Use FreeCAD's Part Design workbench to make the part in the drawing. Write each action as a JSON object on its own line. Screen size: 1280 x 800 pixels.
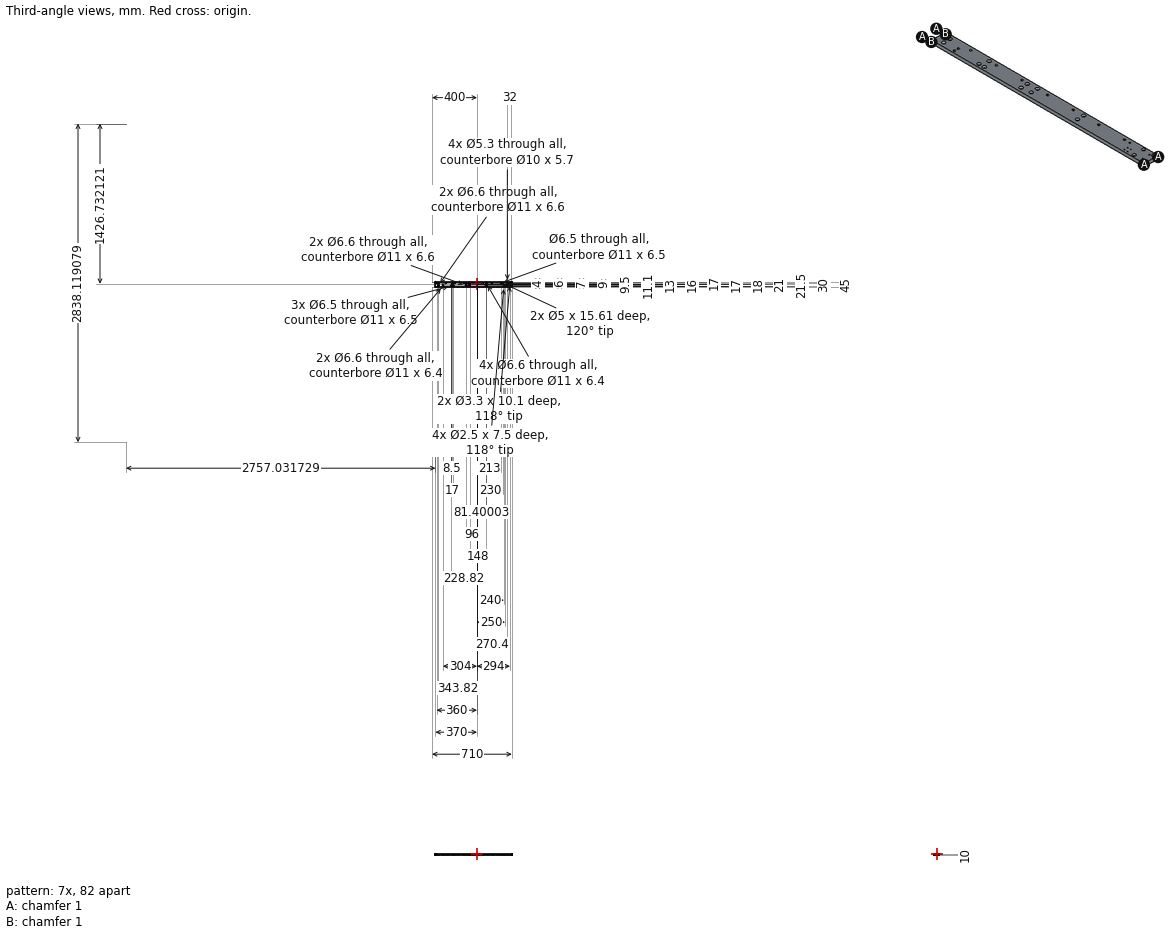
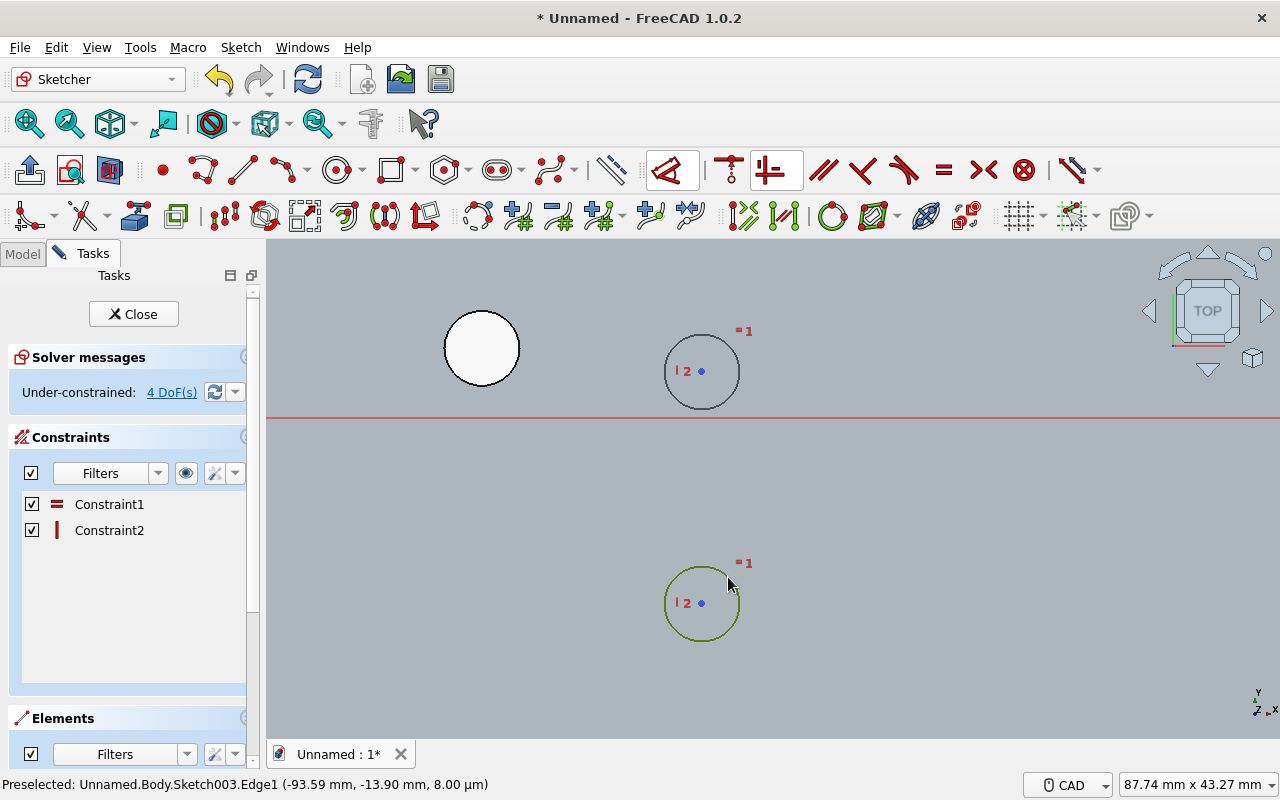
{"action": "key", "text": "k o"}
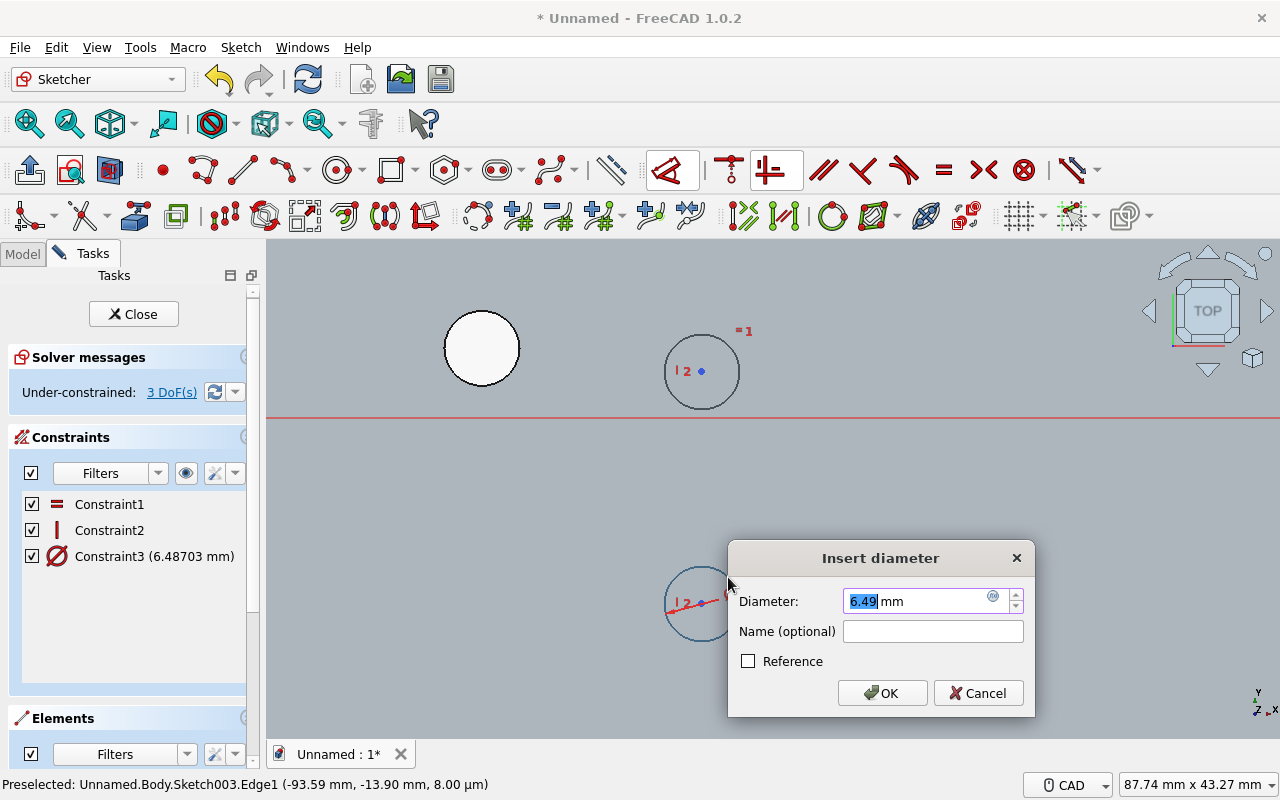
{"action": "type", "text": "6.6"}
{"action": "key", "text": "Return"}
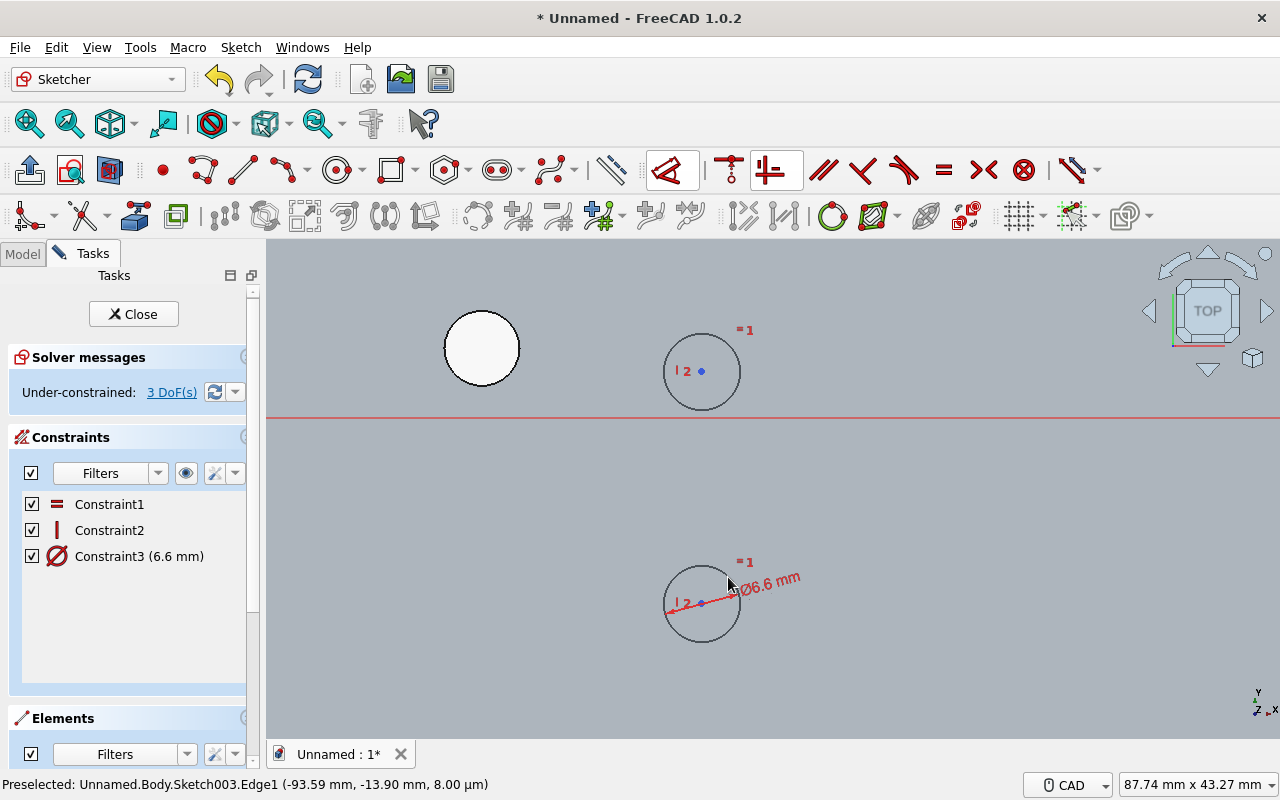
{"action": "left_click", "coordinate": [702, 372]}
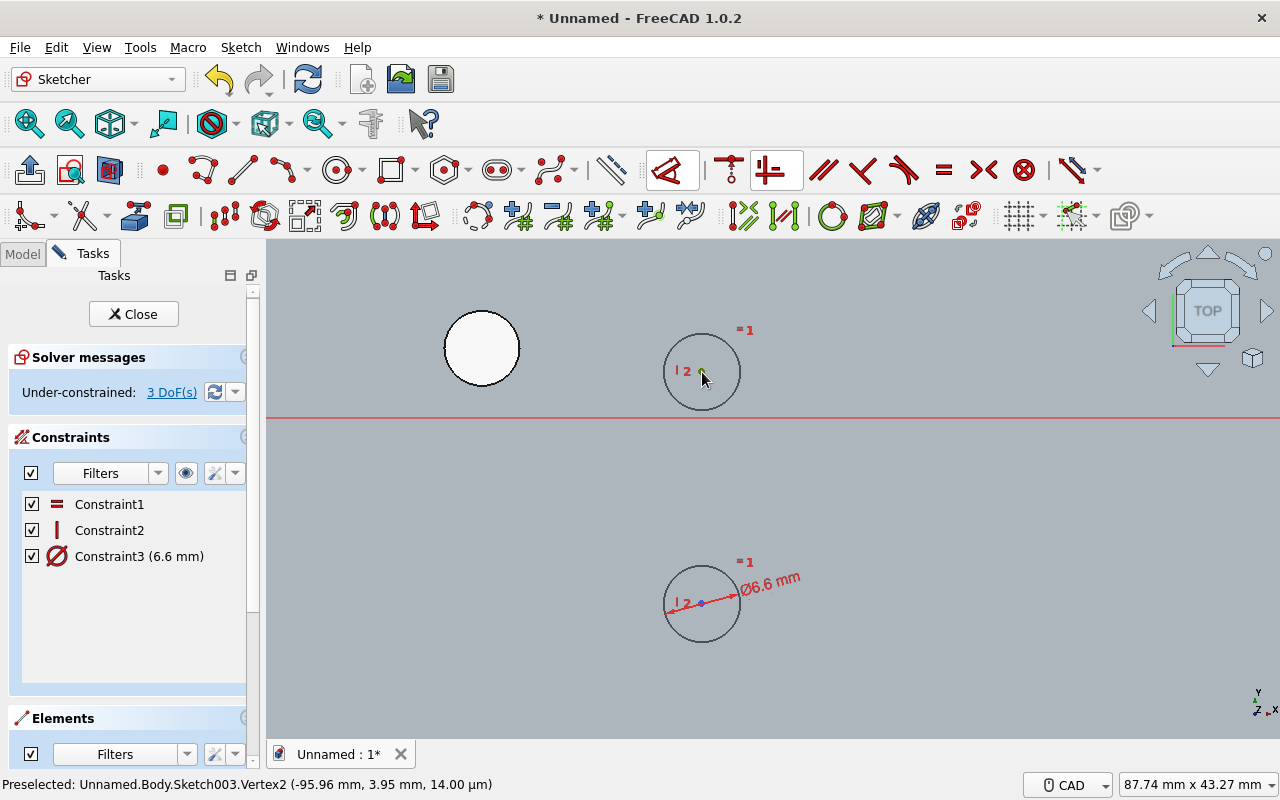
{"action": "key", "text": "i"}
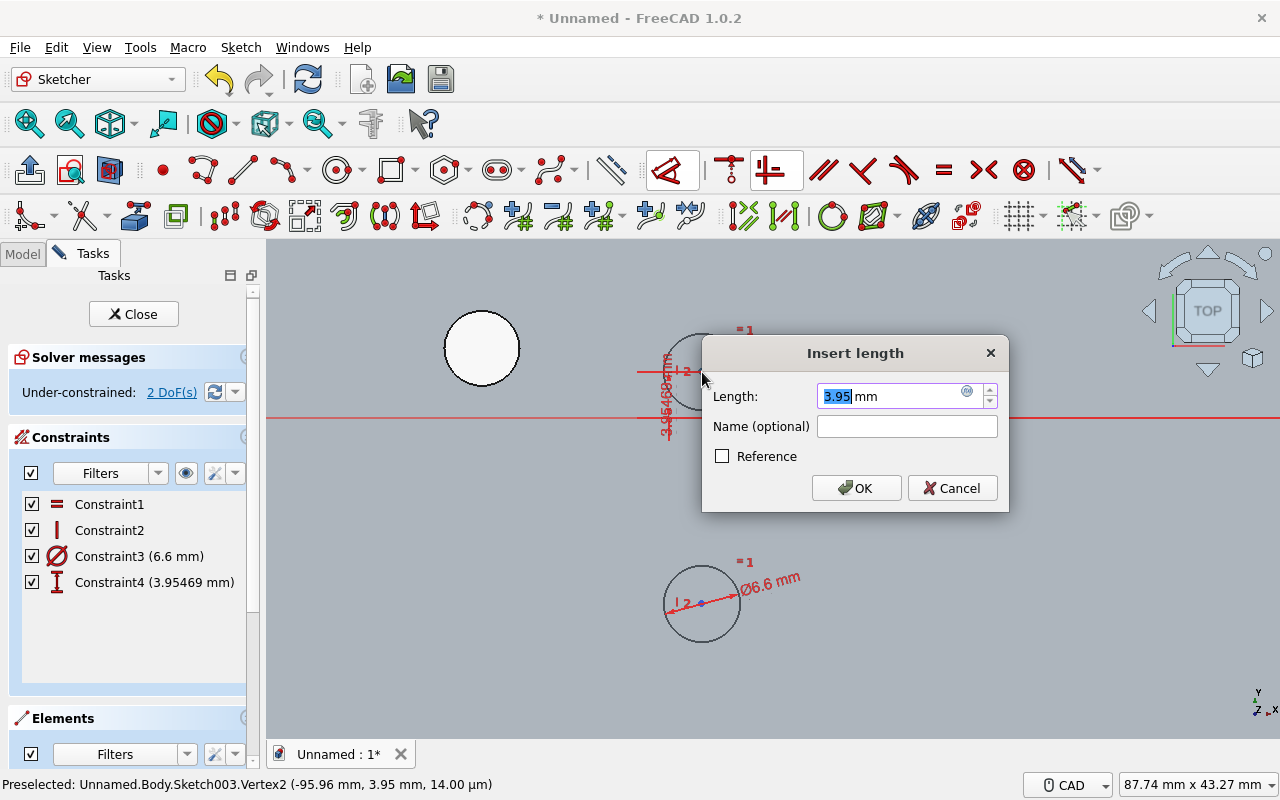
{"action": "type", "text": "4"}
{"action": "key", "text": "Return"}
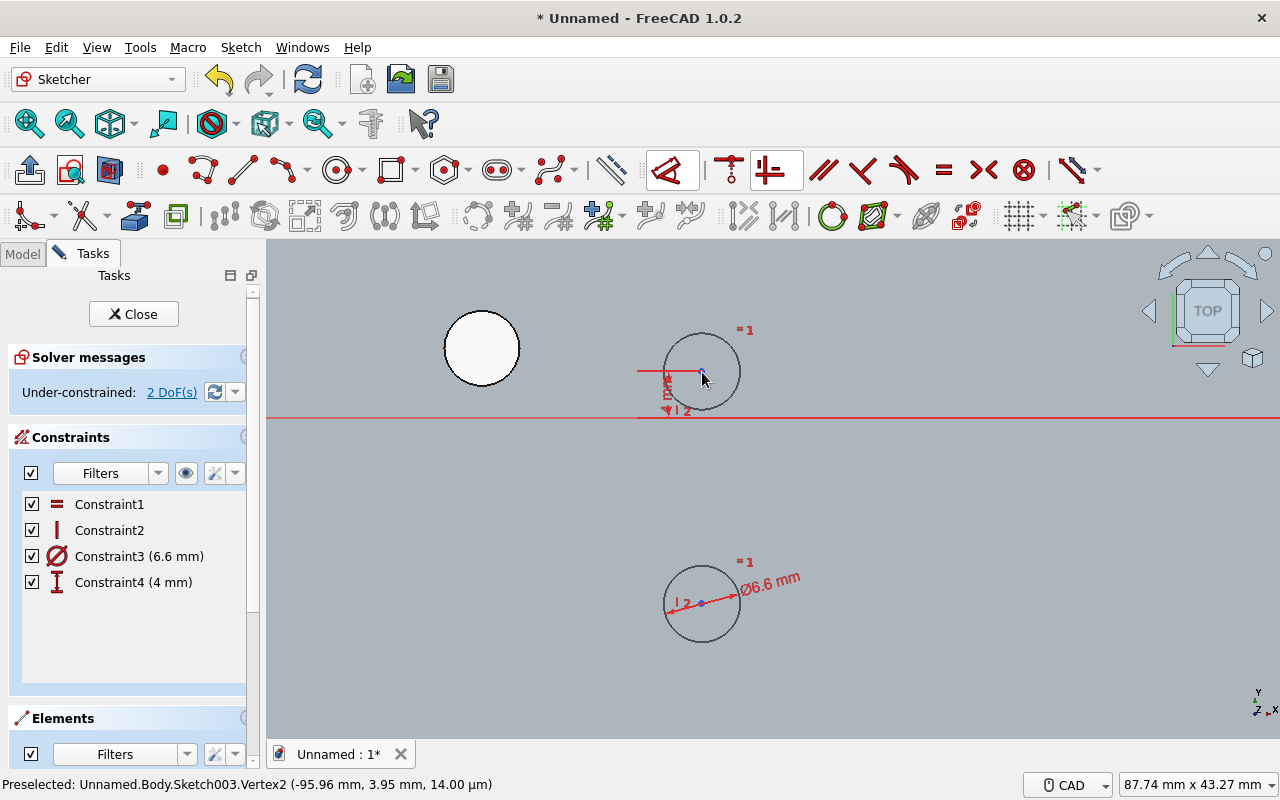
{"action": "left_click", "coordinate": [702, 604]}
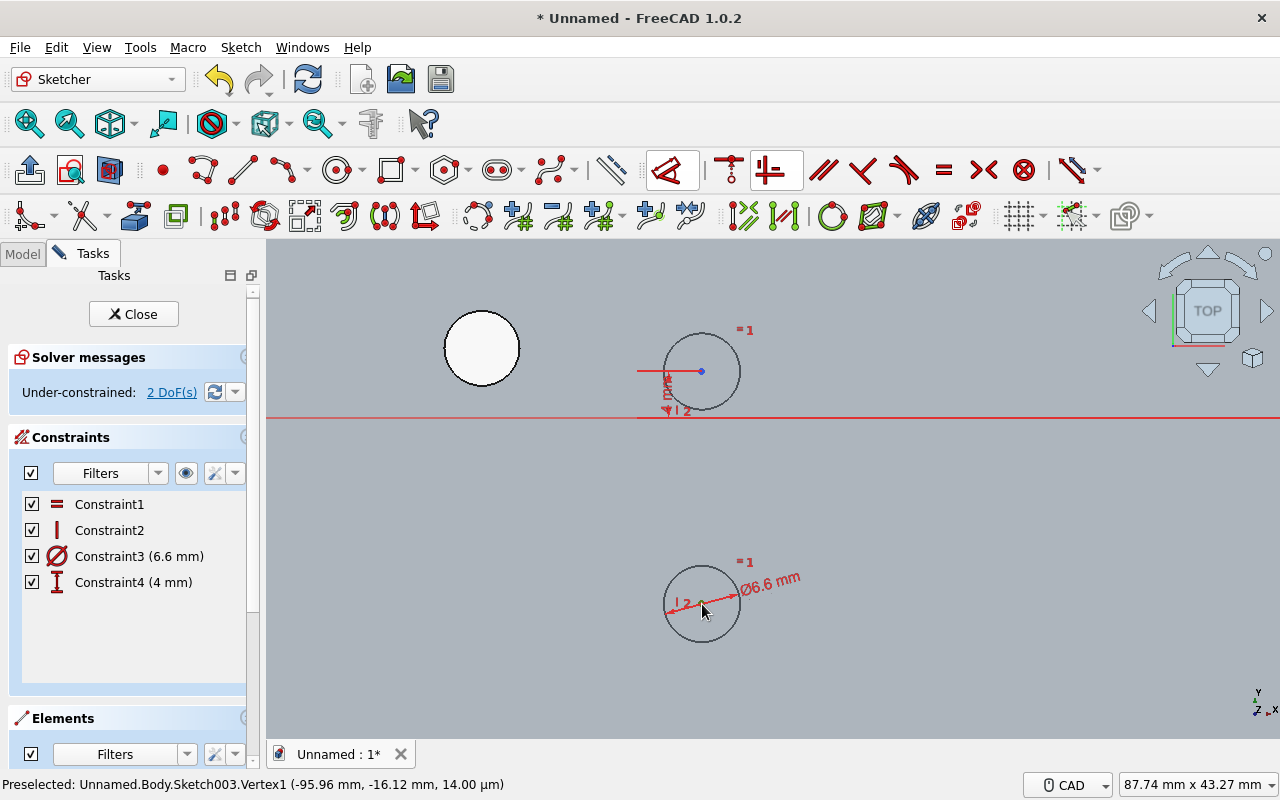
{"action": "left_click", "coordinate": [694, 170]}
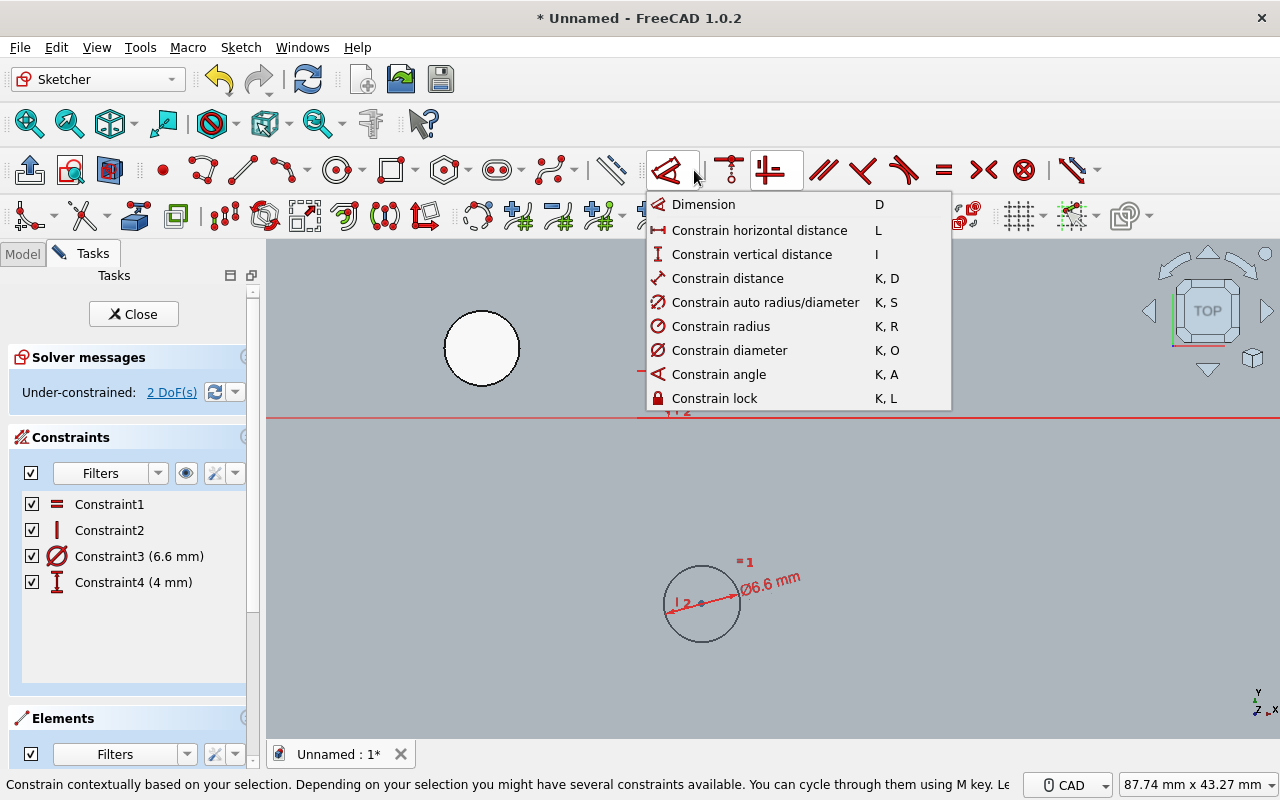
{"action": "left_click", "coordinate": [799, 230]}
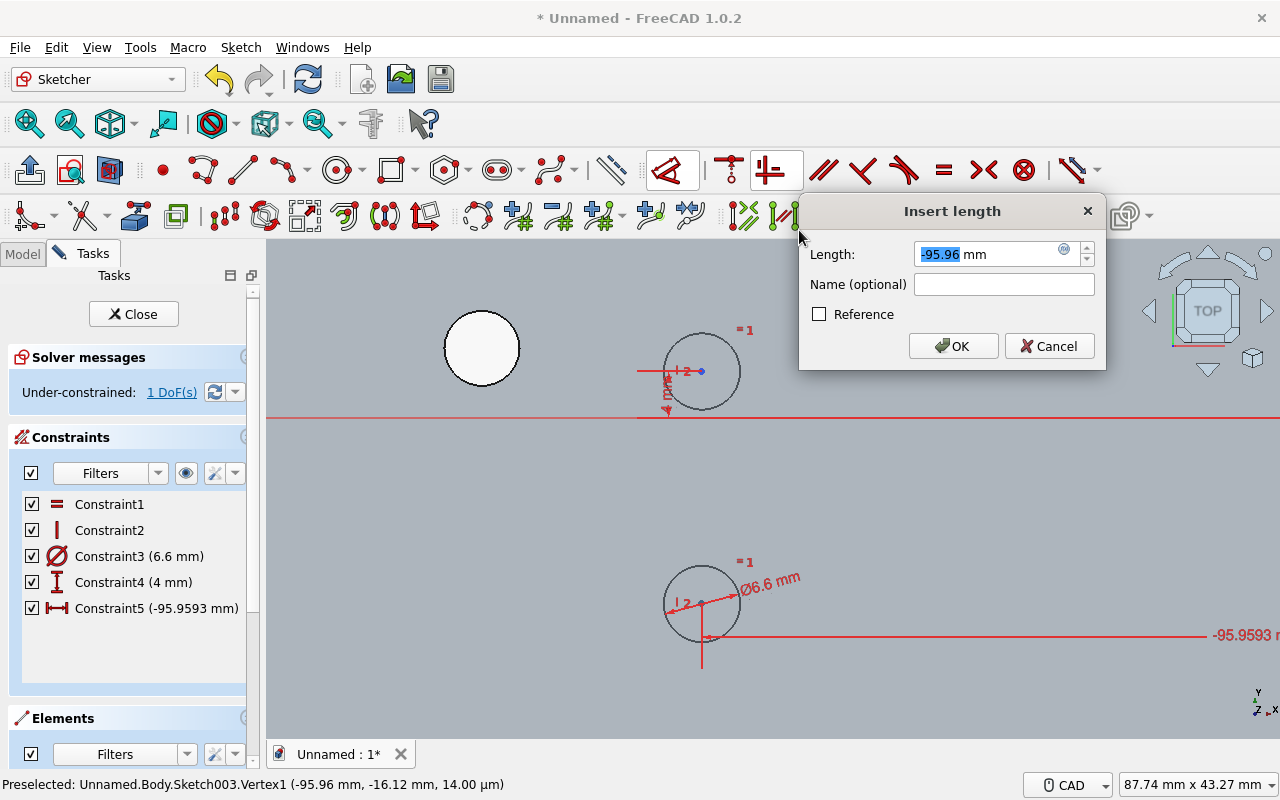
{"action": "type", "text": "-96"}
{"action": "key", "text": "Return"}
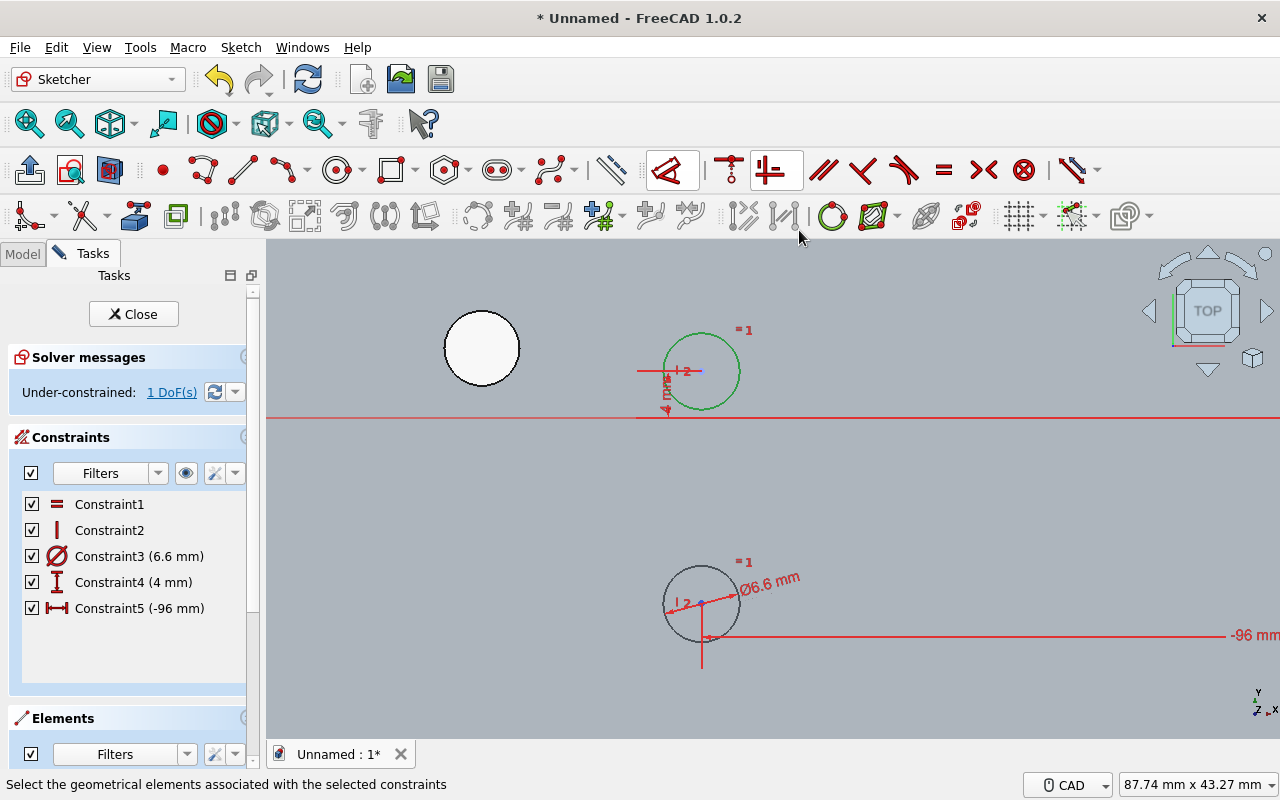
{"action": "left_click", "coordinate": [702, 604]}